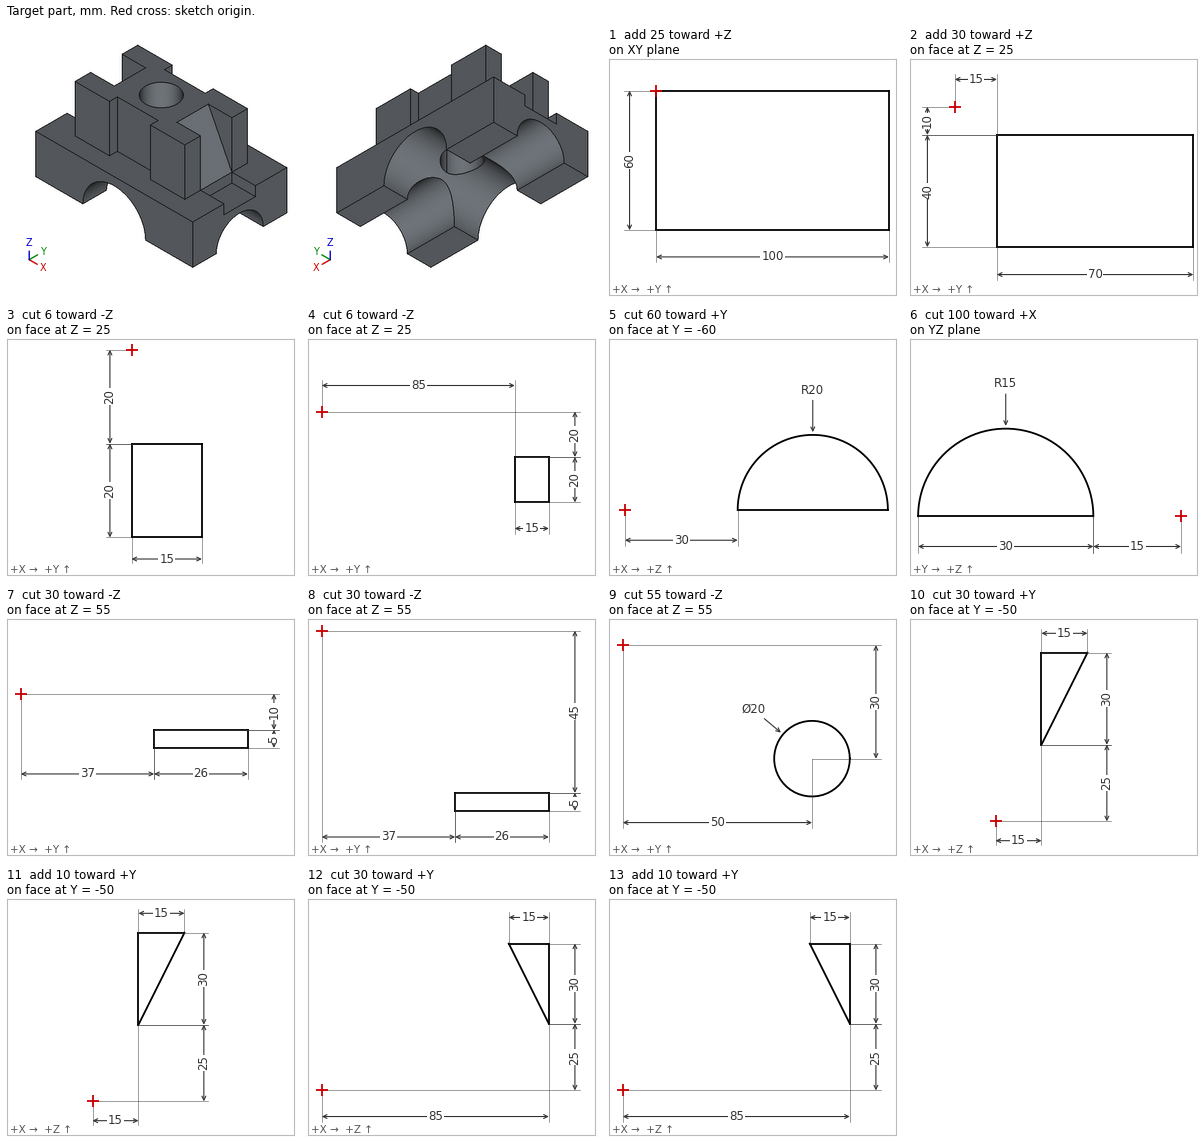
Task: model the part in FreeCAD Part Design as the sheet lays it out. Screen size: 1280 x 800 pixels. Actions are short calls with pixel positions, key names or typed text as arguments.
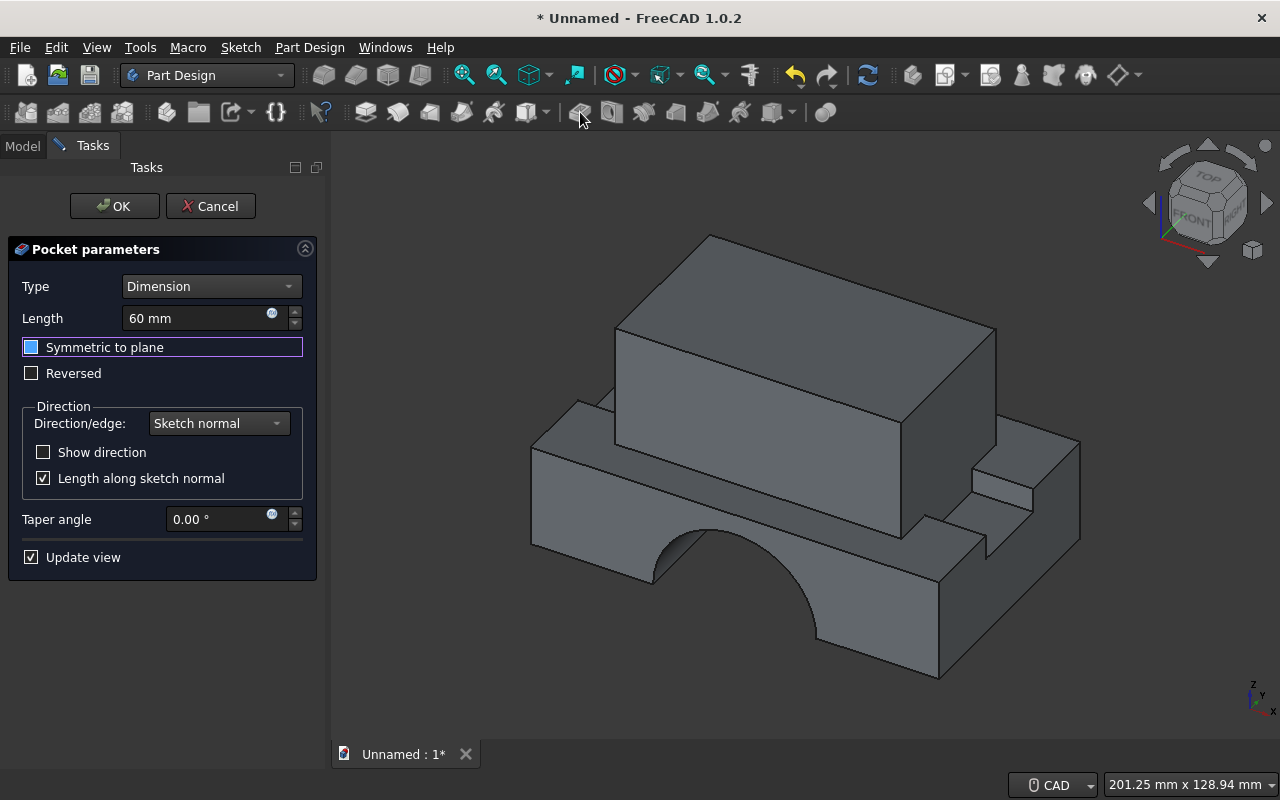
click(115, 206)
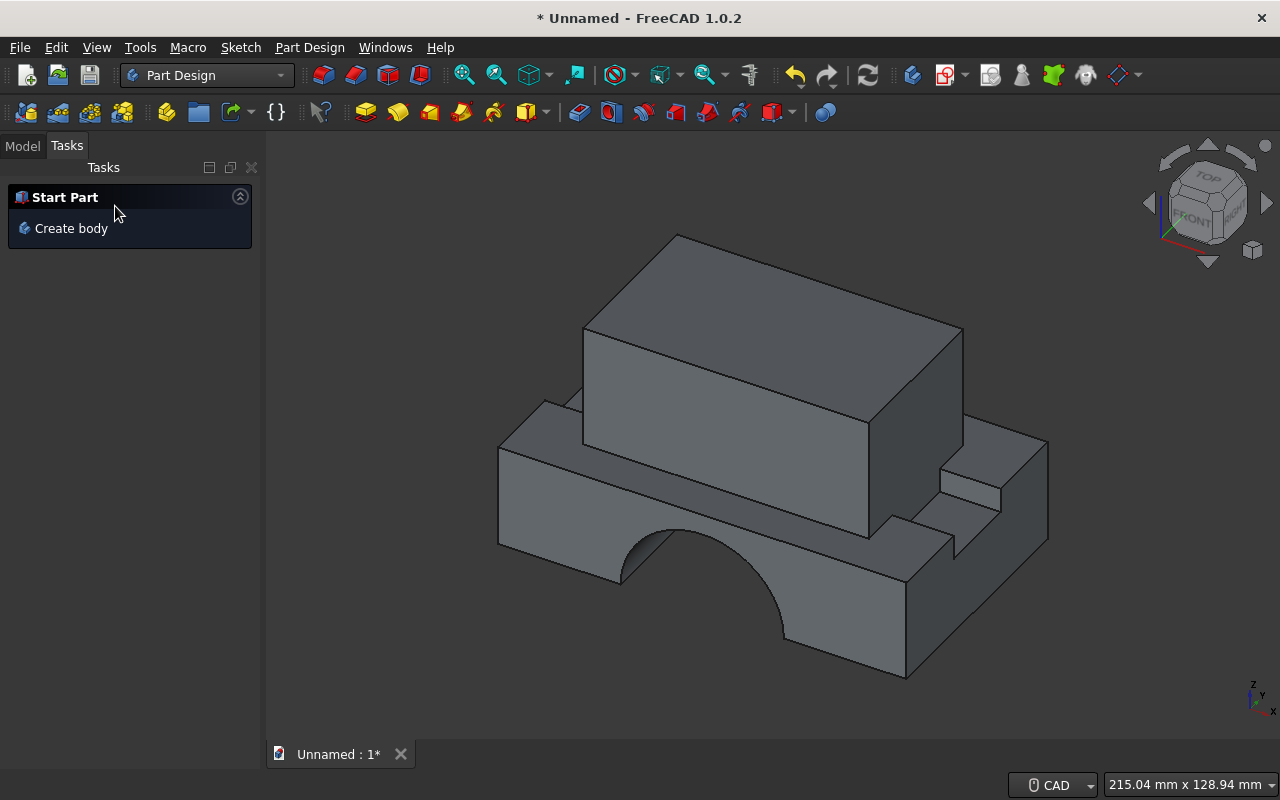
click(946, 76)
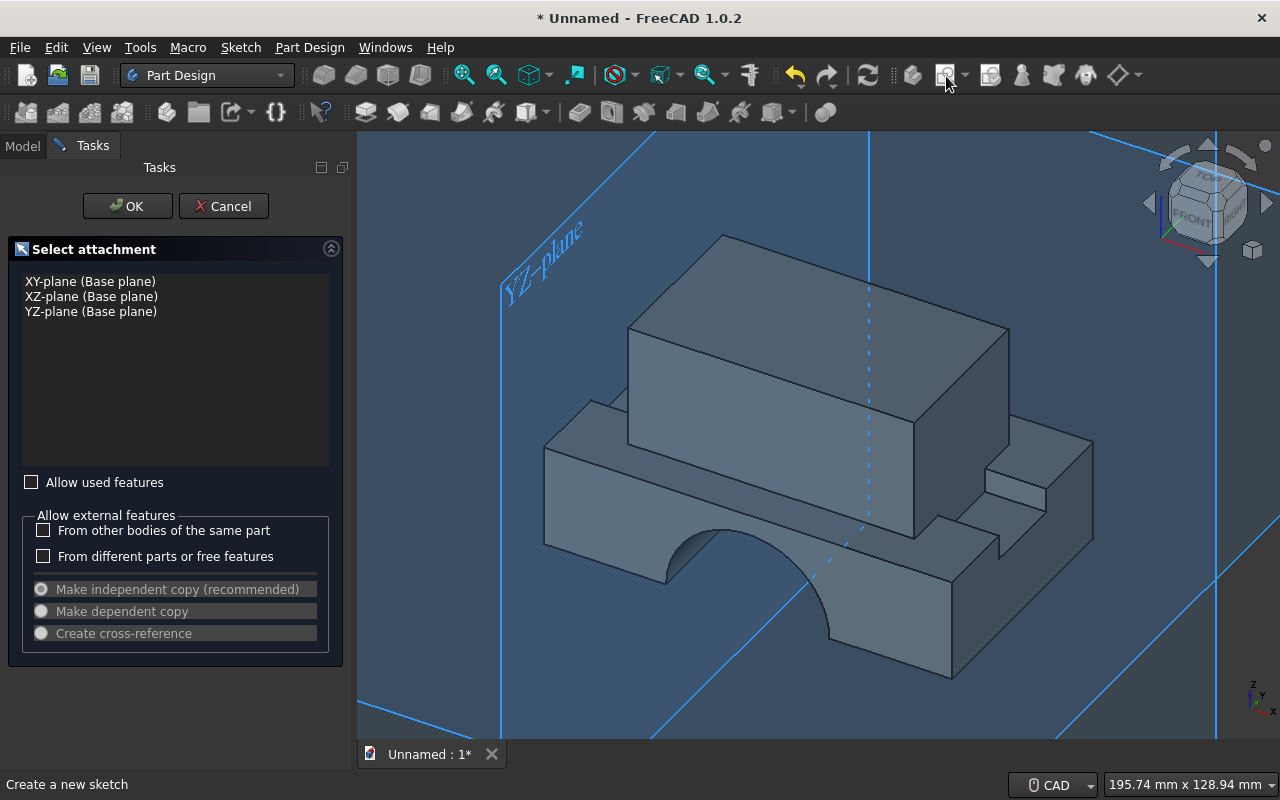
click(82, 312)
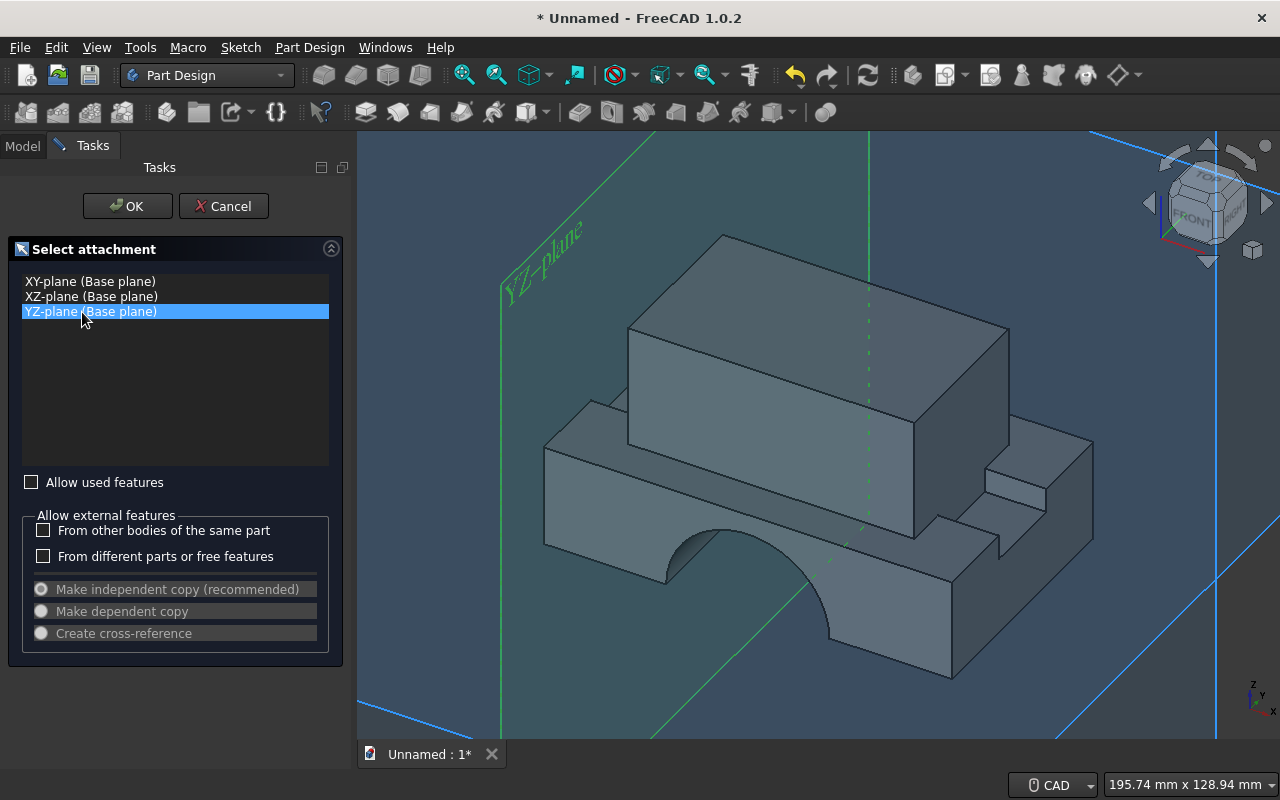
click(128, 206)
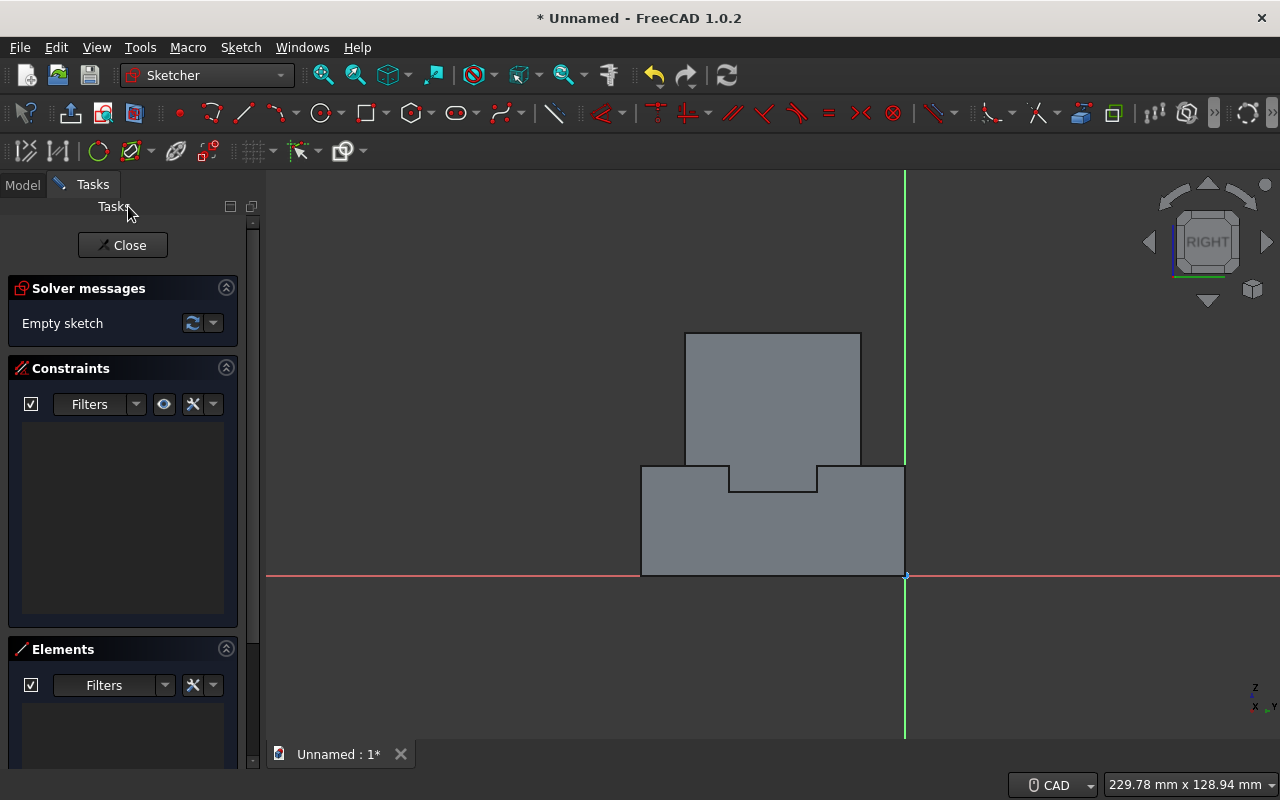
key(q)
key(s)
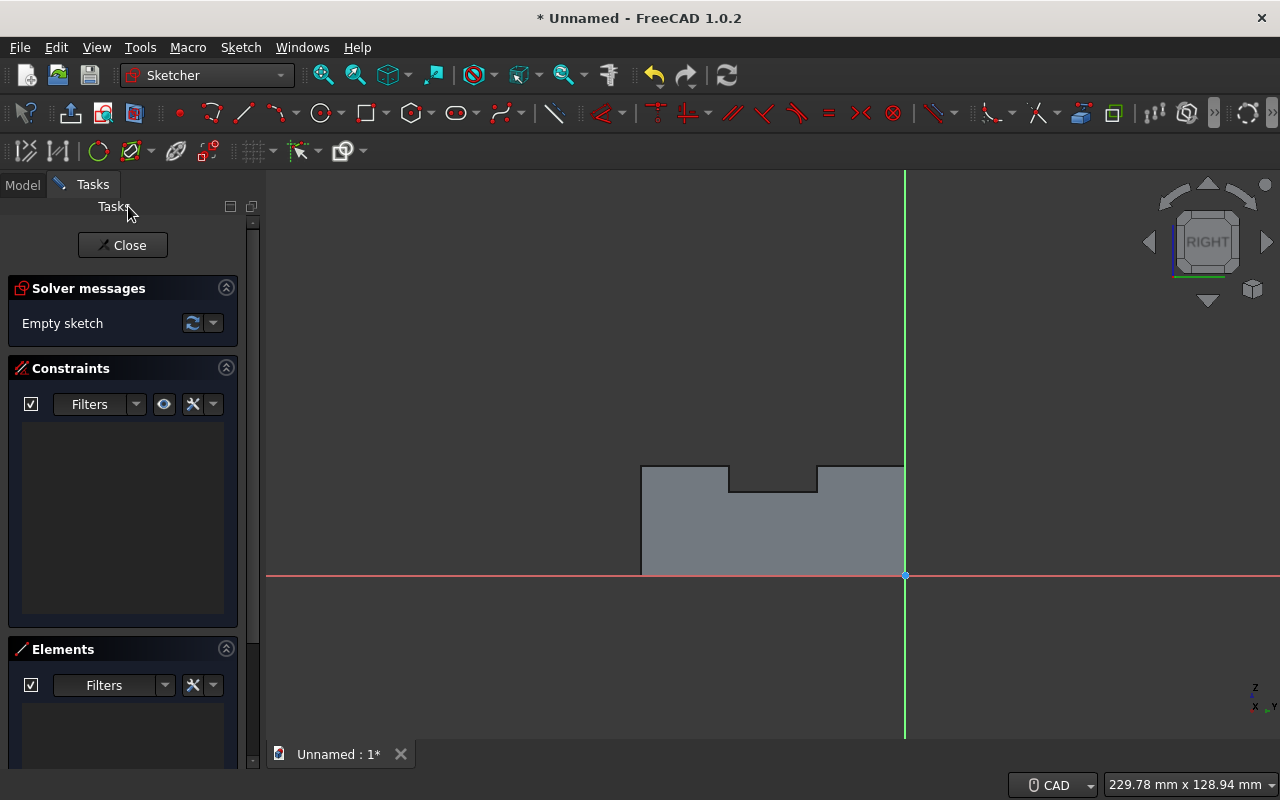
scroll(865, 594, up, 5)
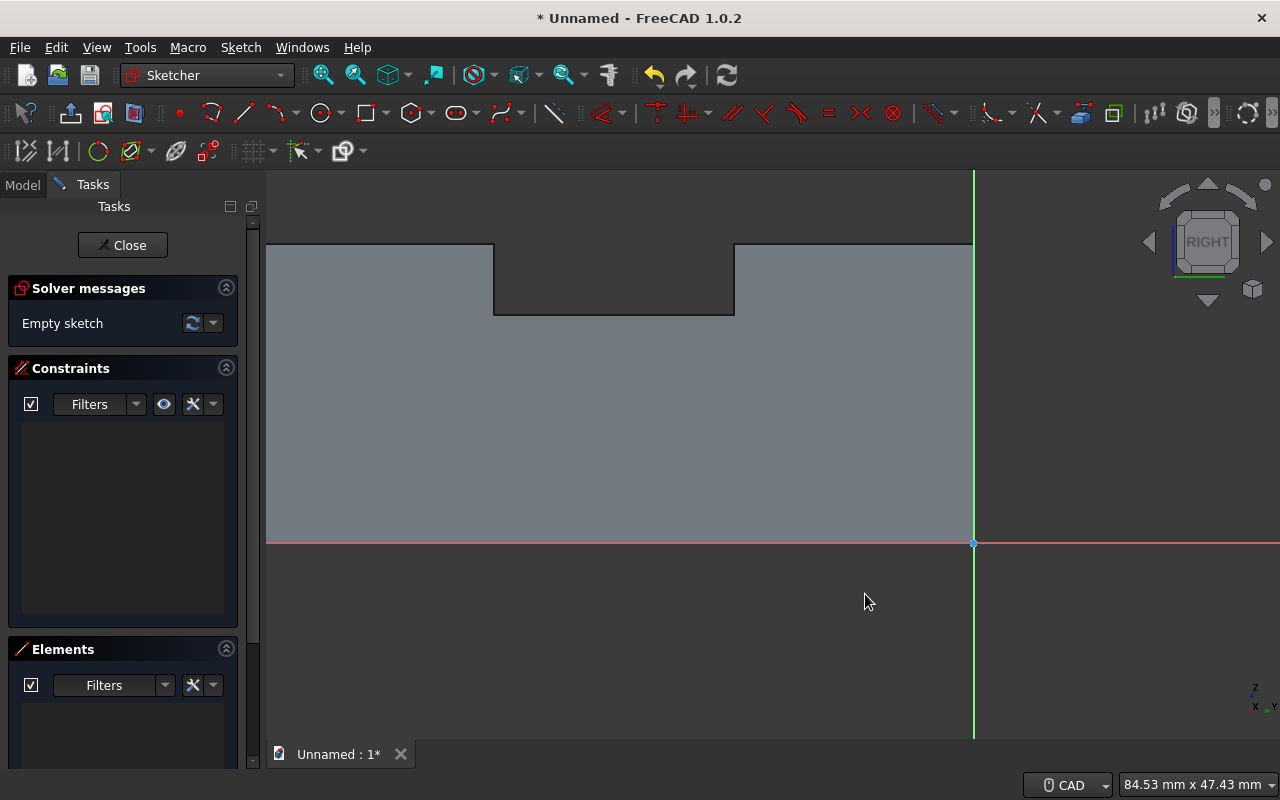
click(244, 114)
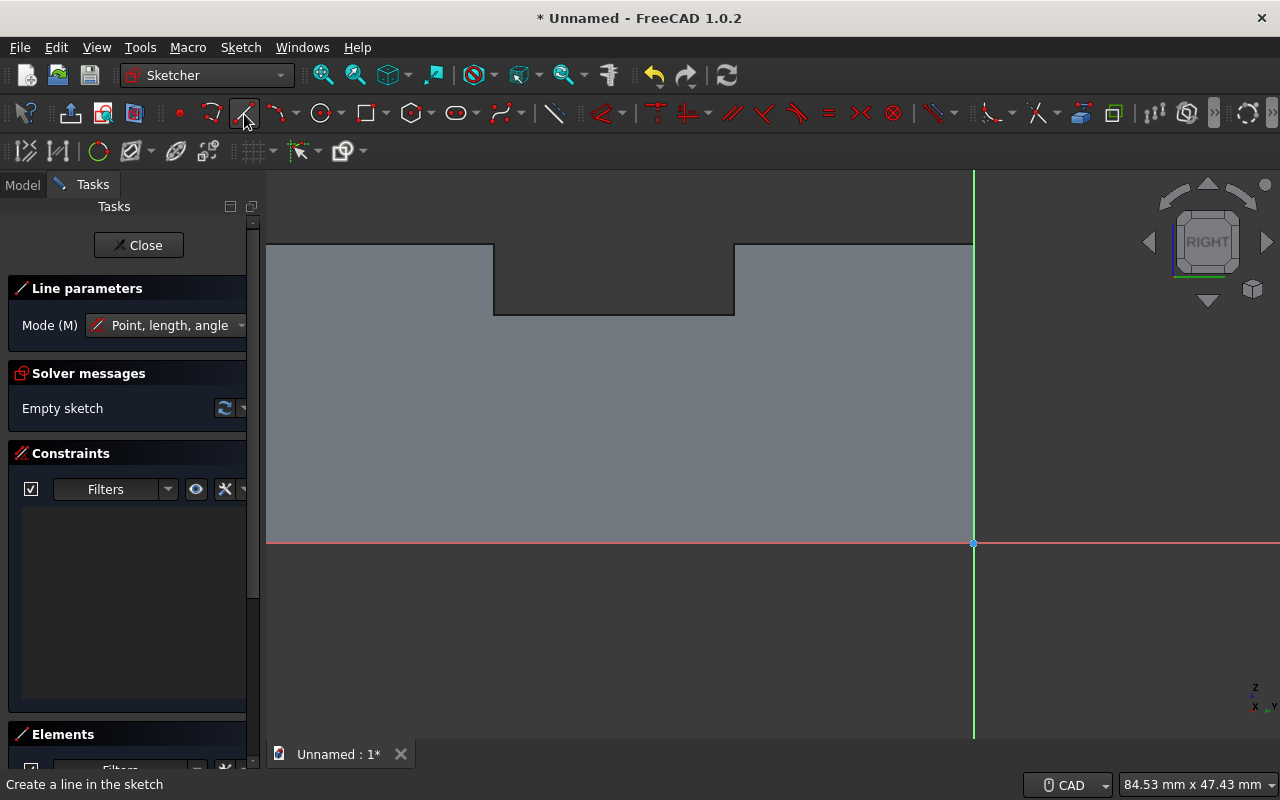
click(794, 543)
click(434, 534)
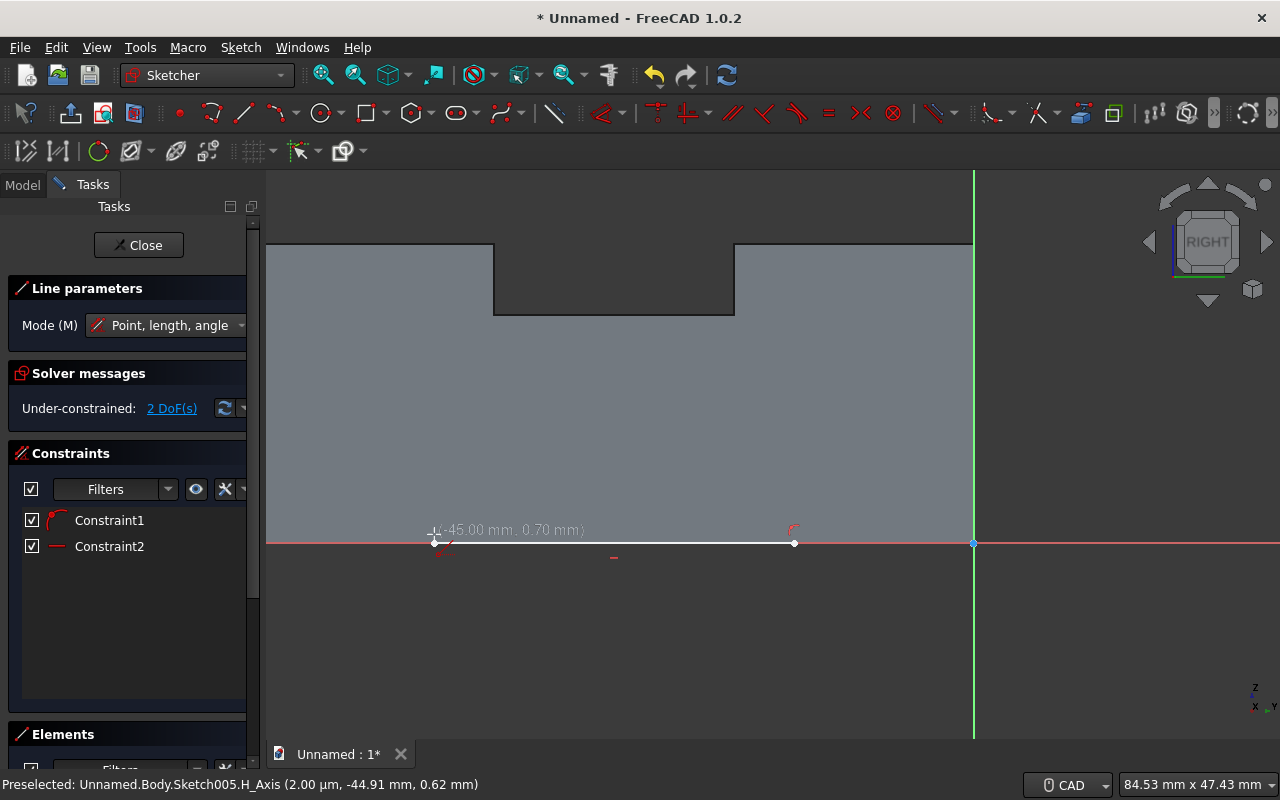
key(g)
key(3)
key(a)